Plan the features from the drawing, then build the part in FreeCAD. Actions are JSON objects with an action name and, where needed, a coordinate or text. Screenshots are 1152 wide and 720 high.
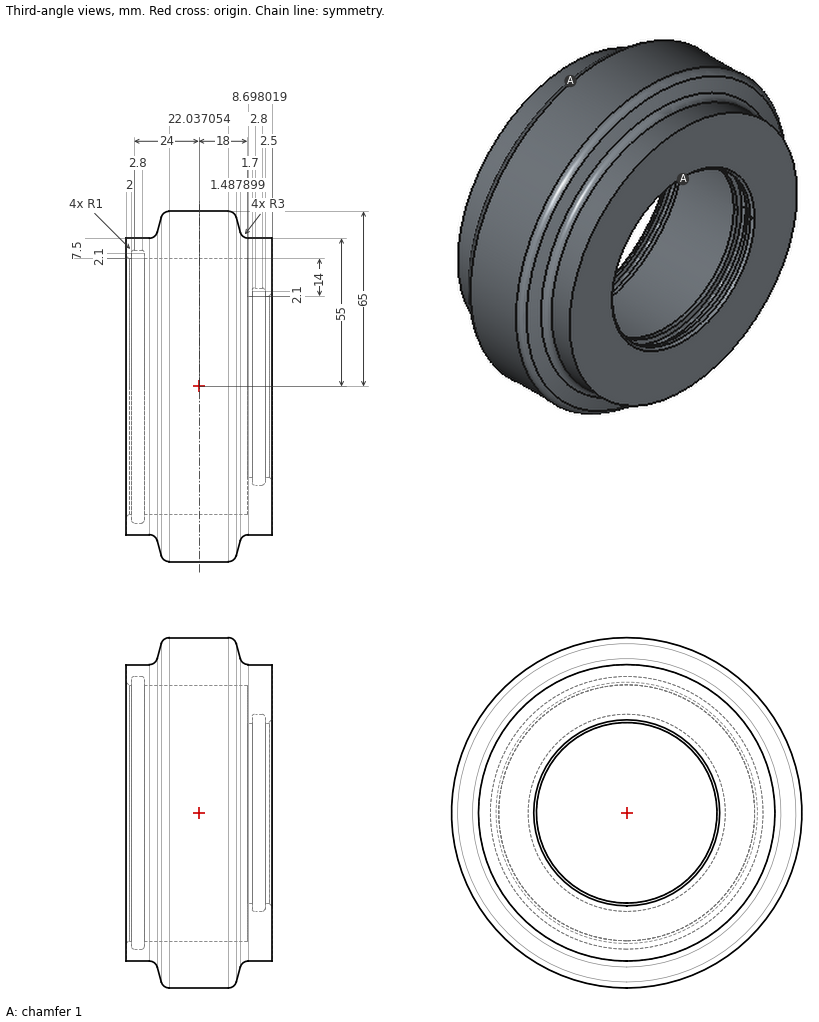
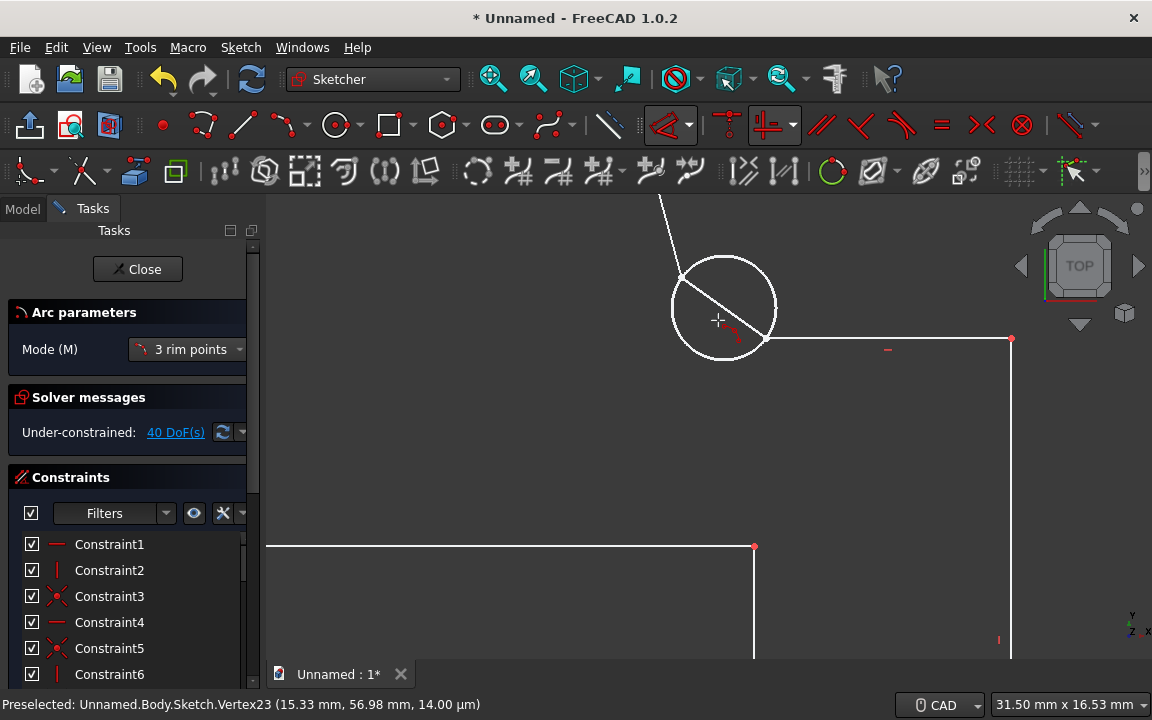
{"action": "left_click", "coordinate": [714, 316]}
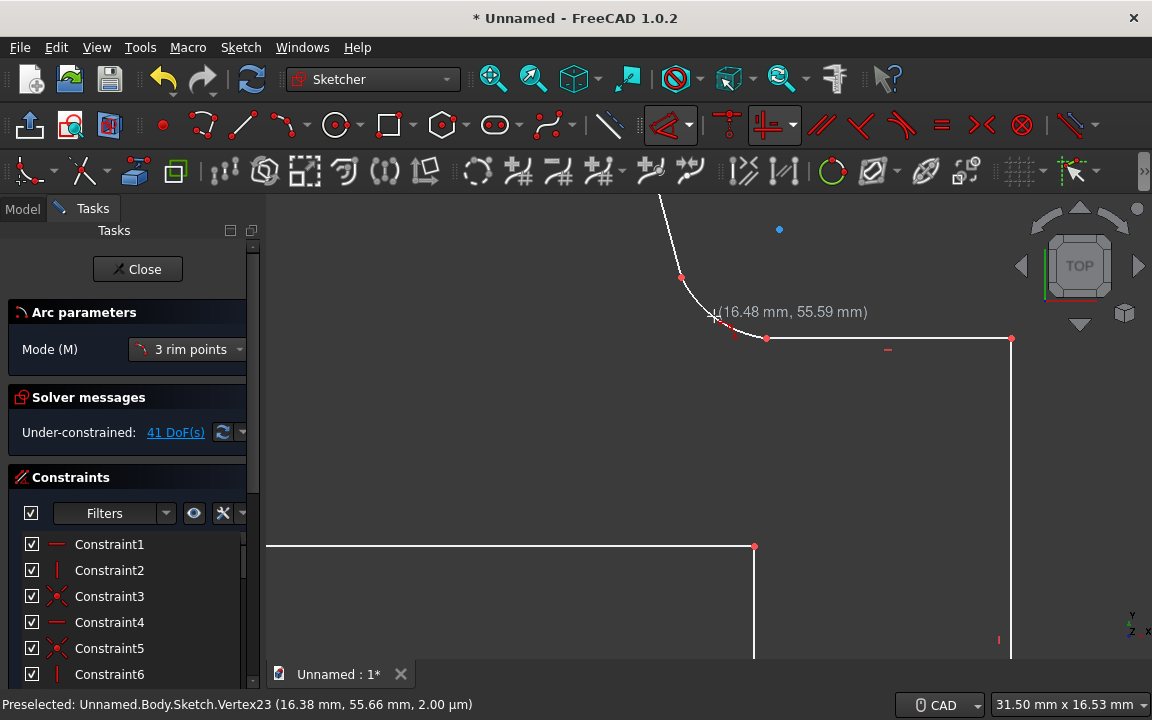
{"action": "scroll", "coordinate": [718, 320], "scroll_direction": "down", "scroll_amount": 9}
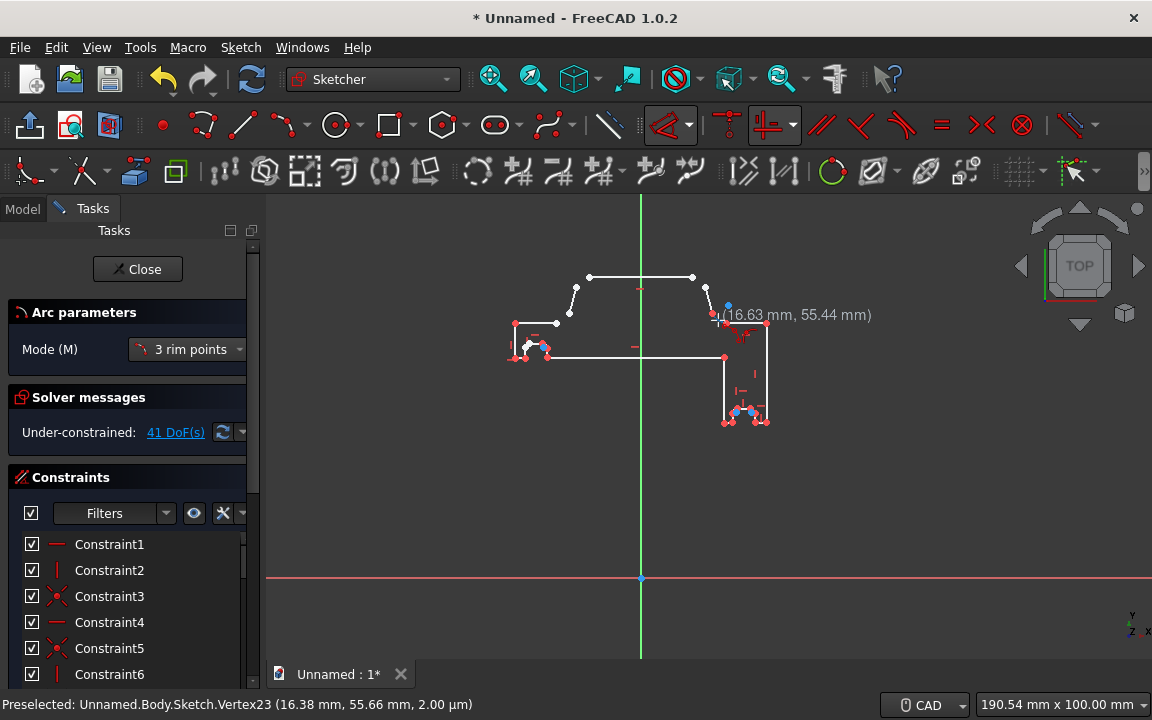
{"action": "left_click", "coordinate": [705, 287]}
{"action": "left_click", "coordinate": [692, 277]}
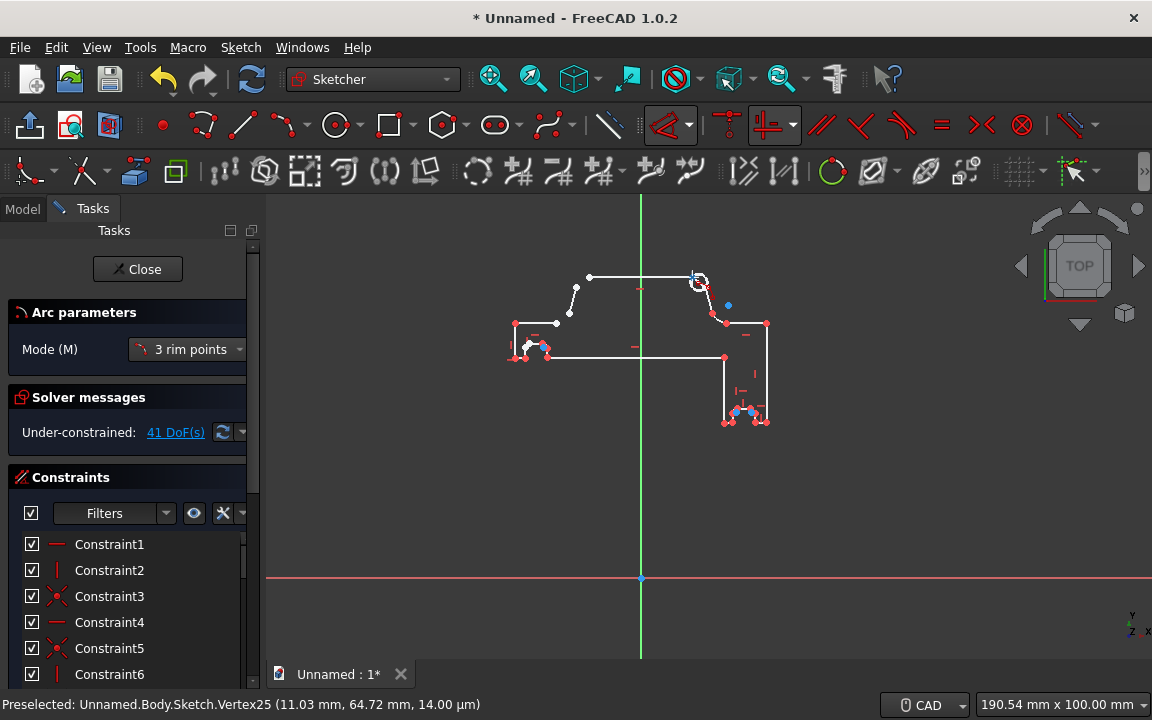
{"action": "scroll", "coordinate": [701, 279], "scroll_direction": "up", "scroll_amount": 9}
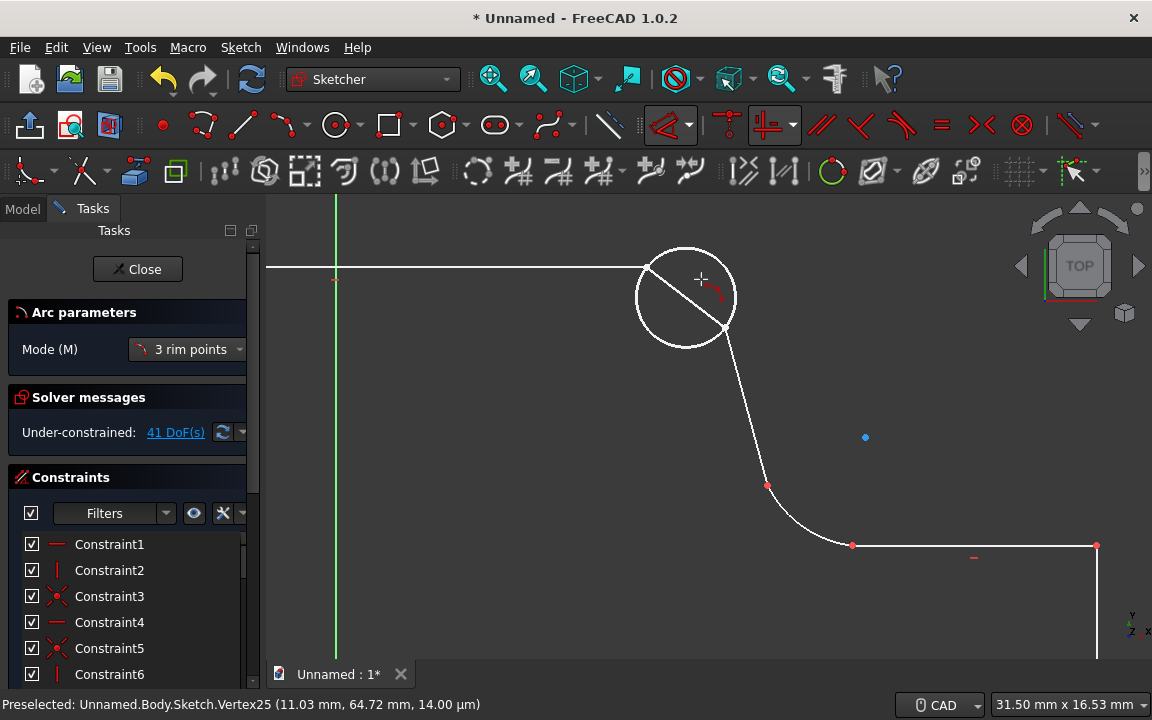
{"action": "left_click", "coordinate": [698, 277]}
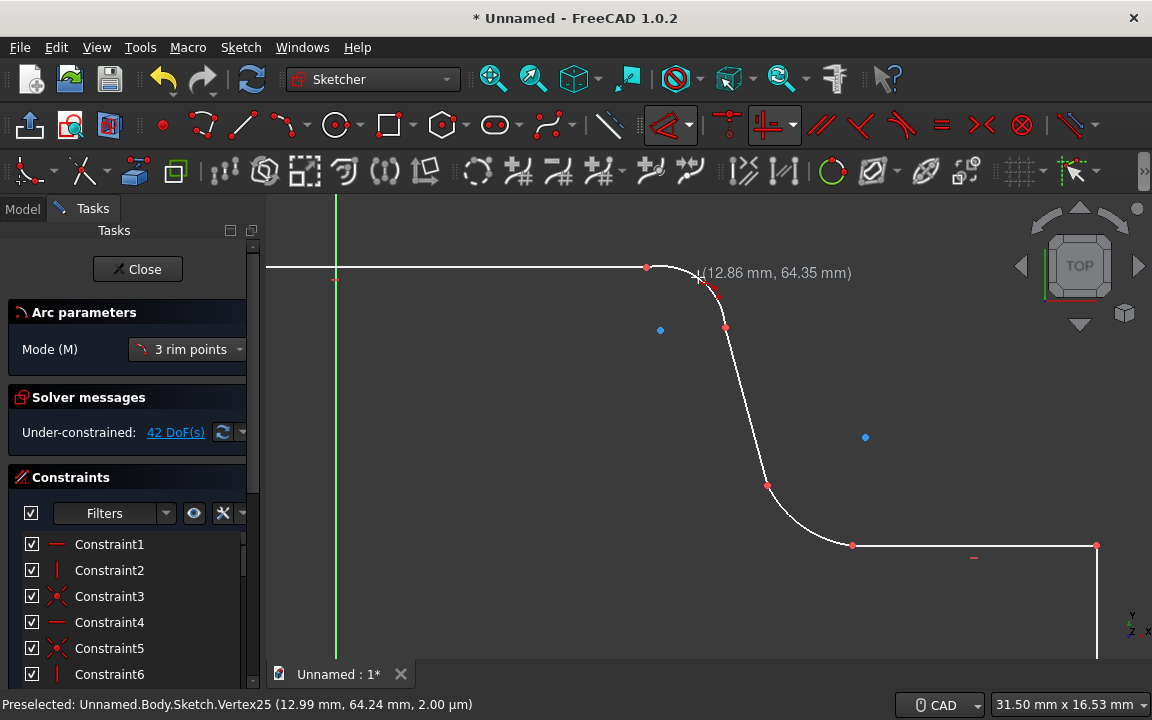
{"action": "scroll", "coordinate": [701, 278], "scroll_direction": "down", "scroll_amount": 9}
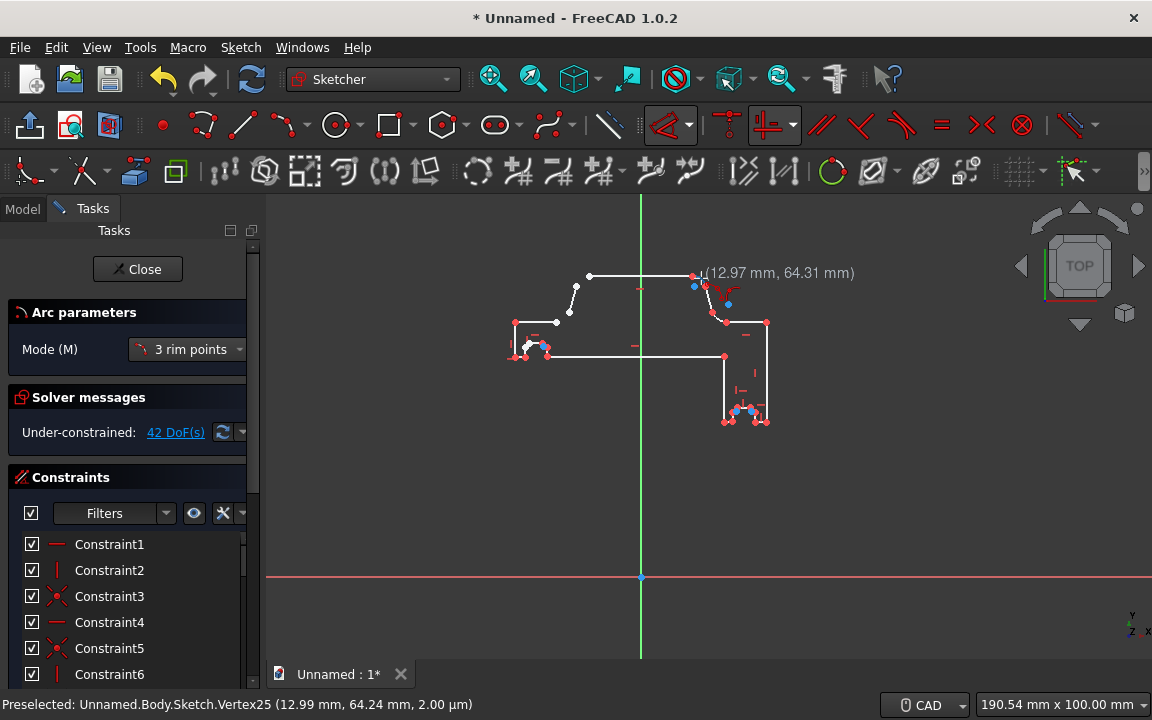
{"action": "left_click", "coordinate": [589, 276]}
{"action": "left_click", "coordinate": [576, 286]}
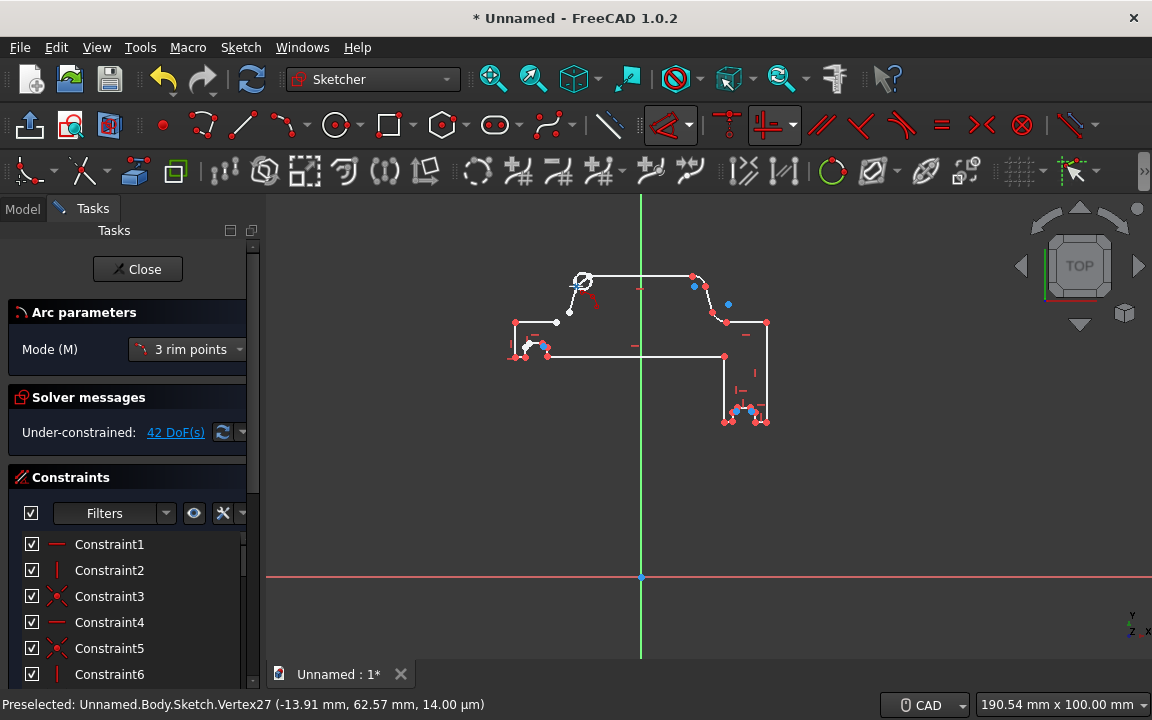
{"action": "scroll", "coordinate": [581, 278], "scroll_direction": "up", "scroll_amount": 9}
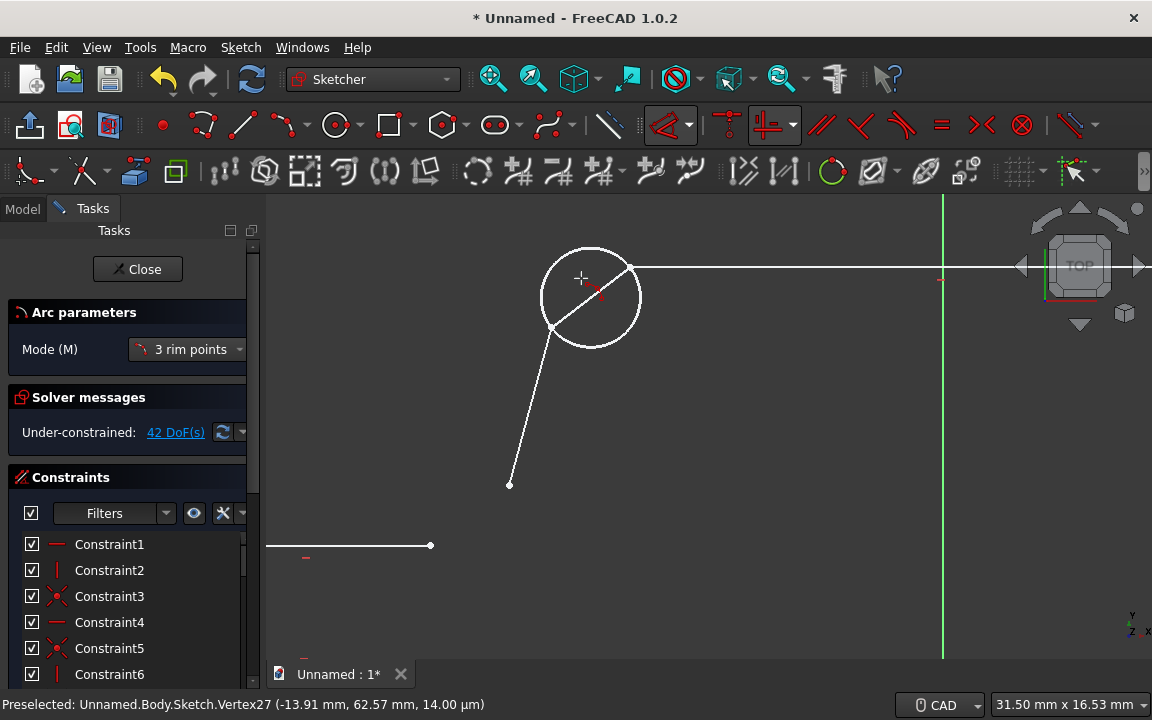
{"action": "left_click", "coordinate": [582, 277]}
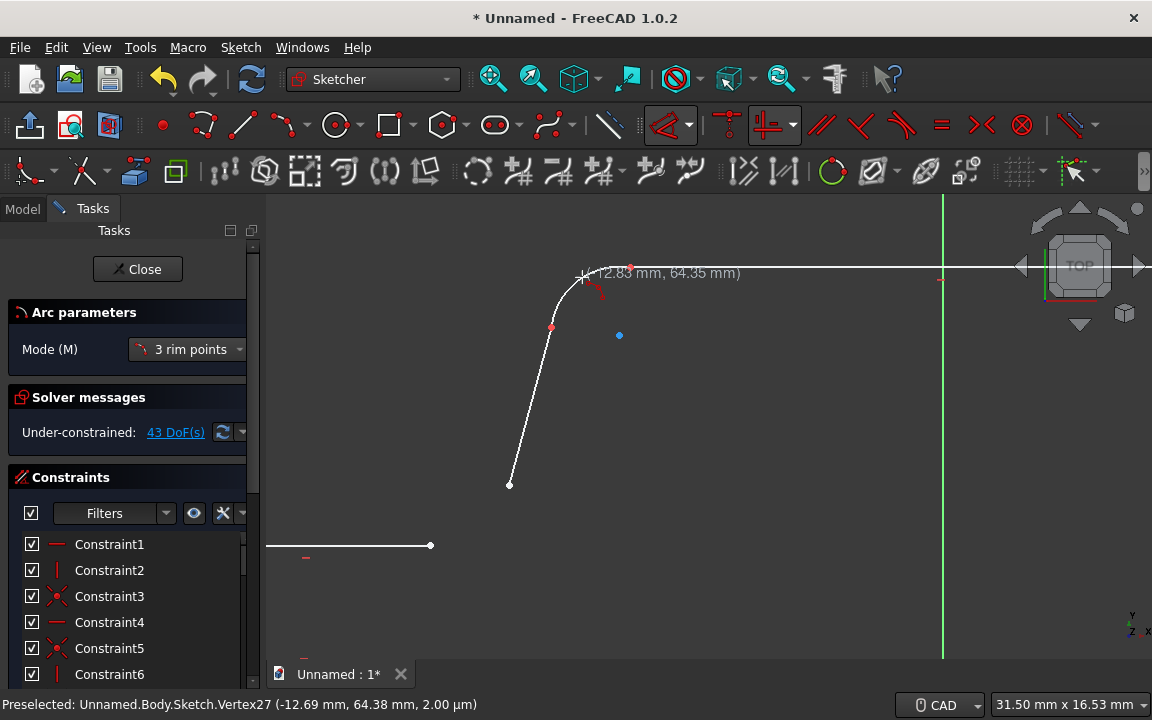
{"action": "scroll", "coordinate": [581, 278], "scroll_direction": "down", "scroll_amount": 9}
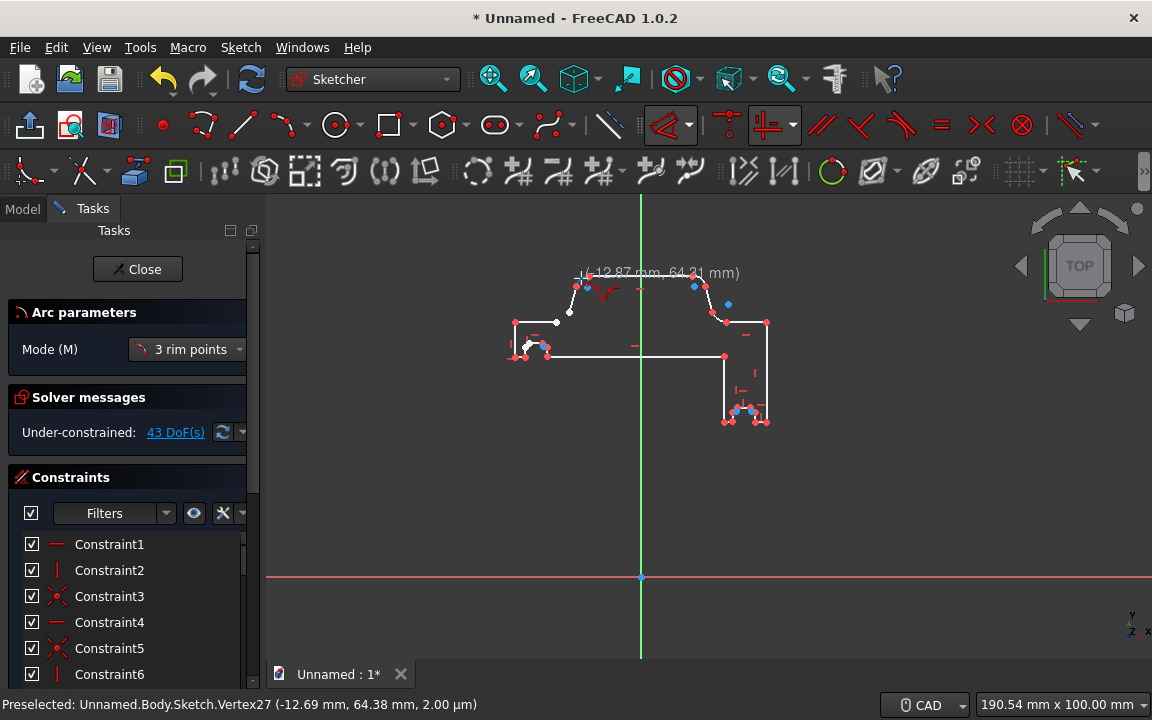
{"action": "left_click", "coordinate": [569, 312]}
{"action": "left_click", "coordinate": [556, 322]}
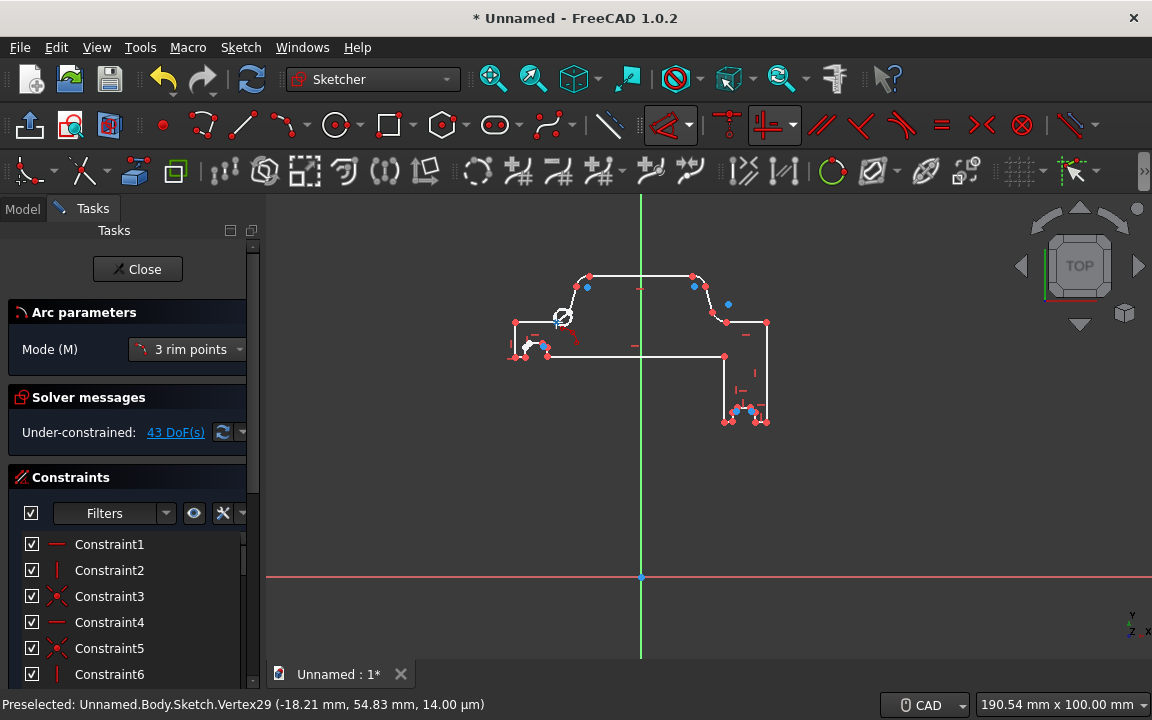
{"action": "scroll", "coordinate": [565, 319], "scroll_direction": "up", "scroll_amount": 9}